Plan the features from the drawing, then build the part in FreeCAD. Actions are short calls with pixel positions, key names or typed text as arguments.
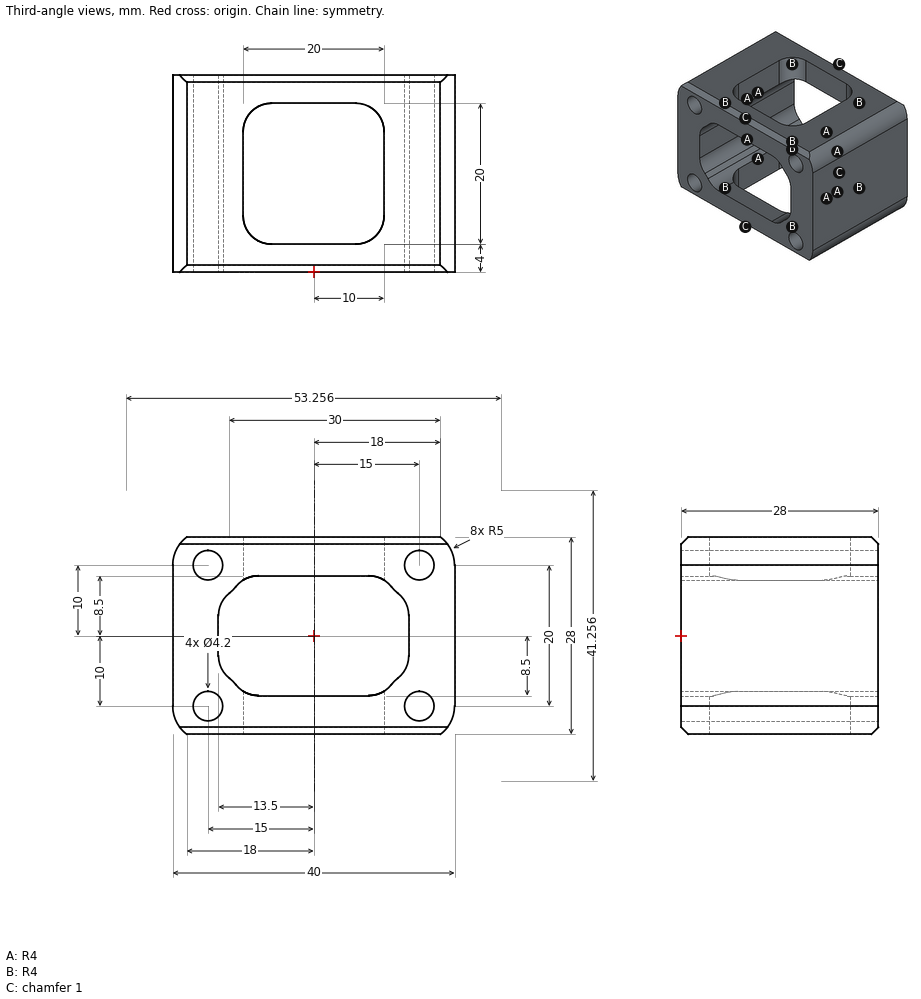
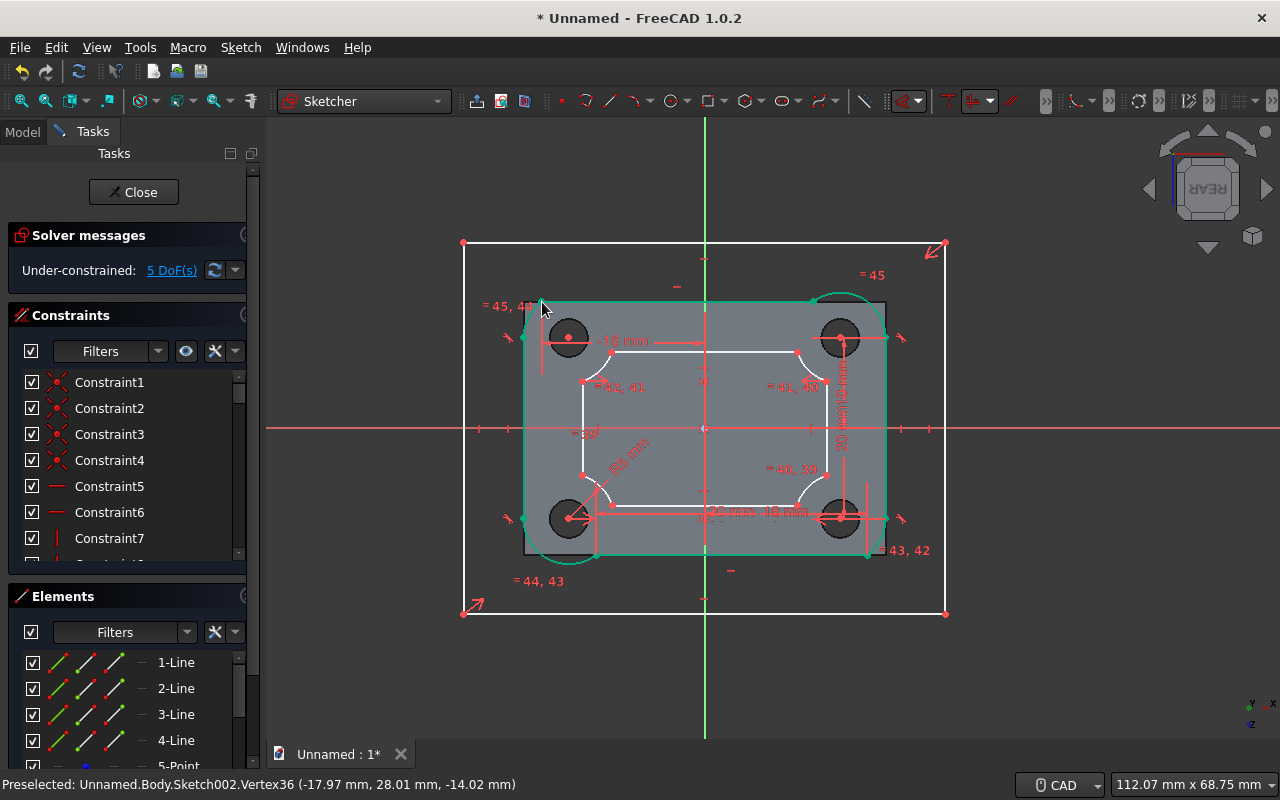
click(612, 506)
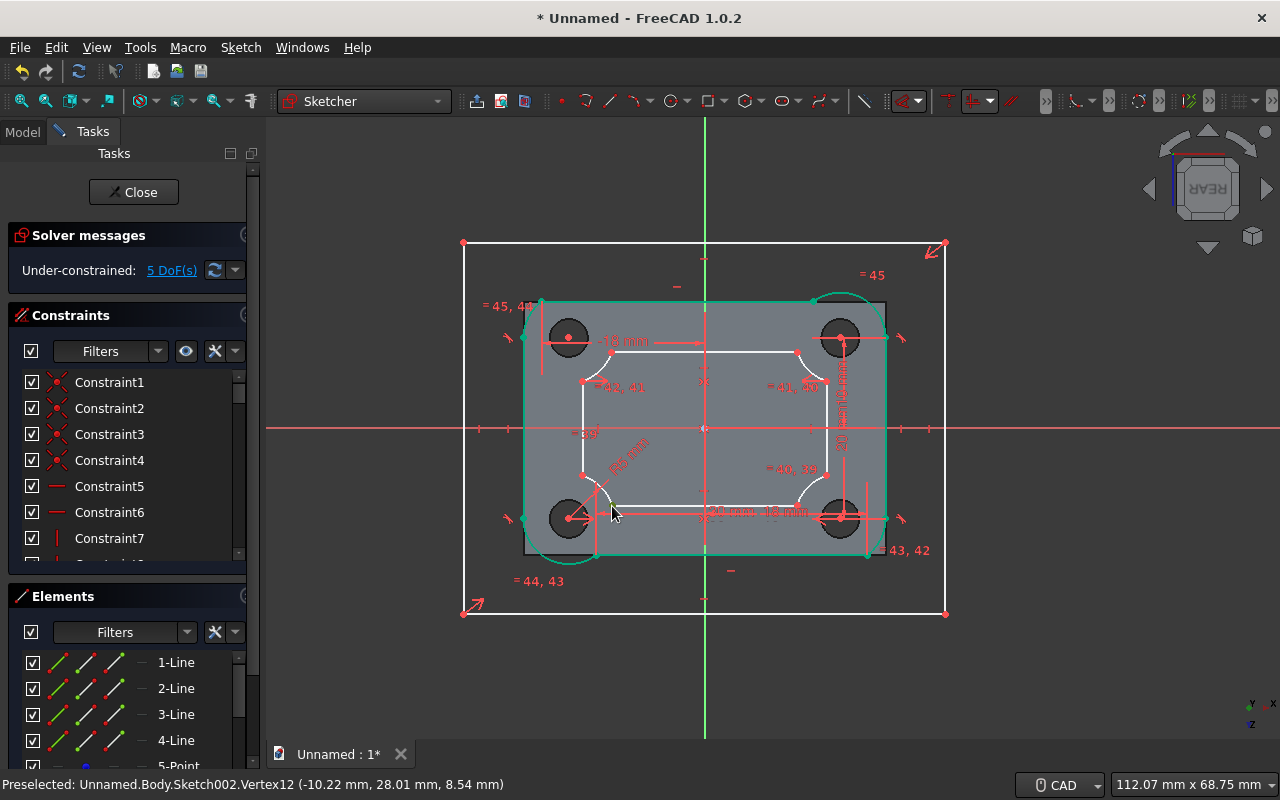
click(920, 102)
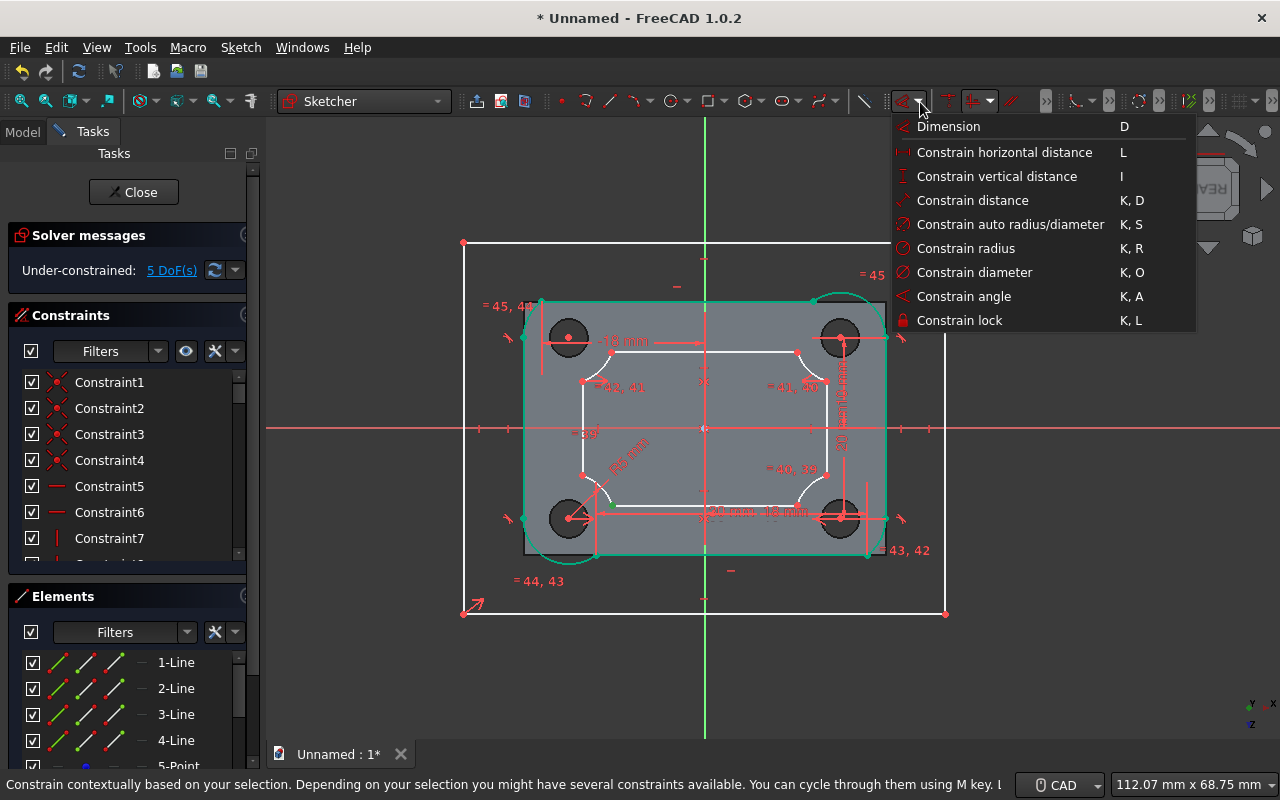
click(1044, 176)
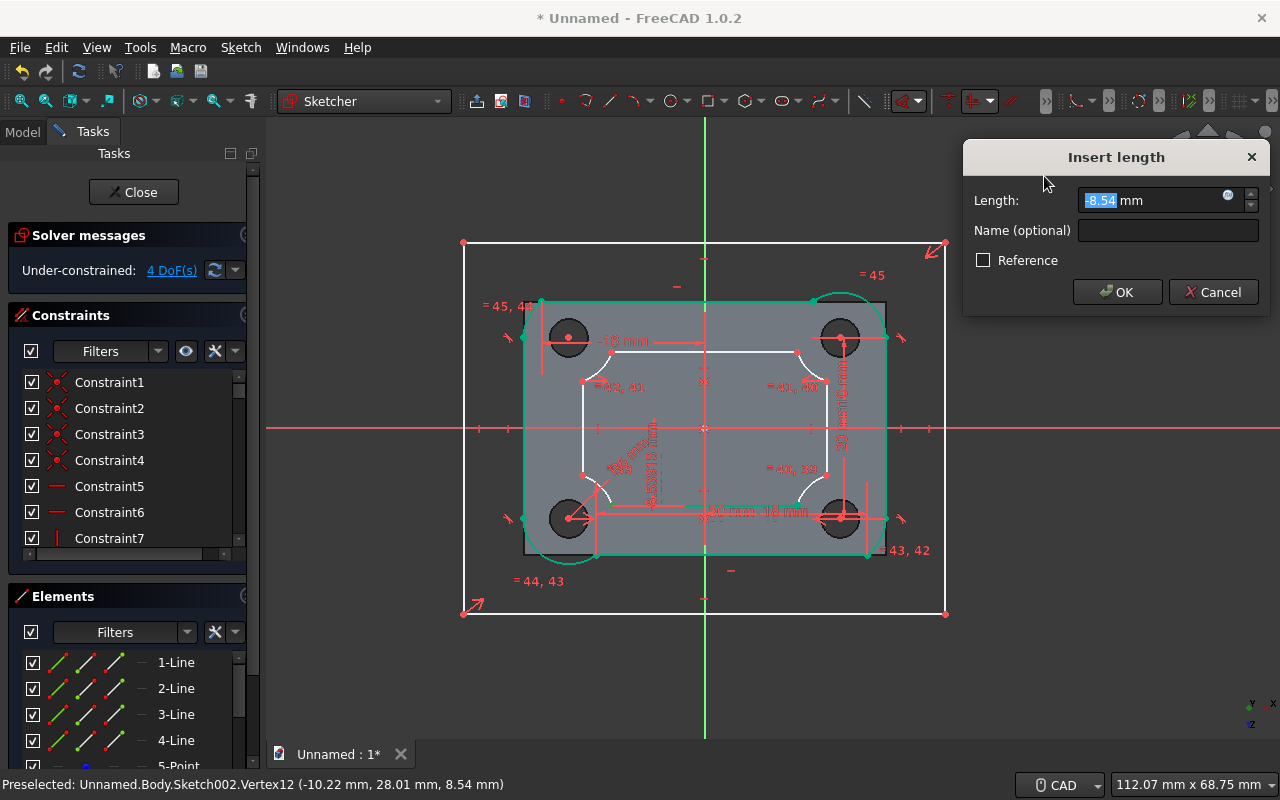
text(-8.5)
key(Return)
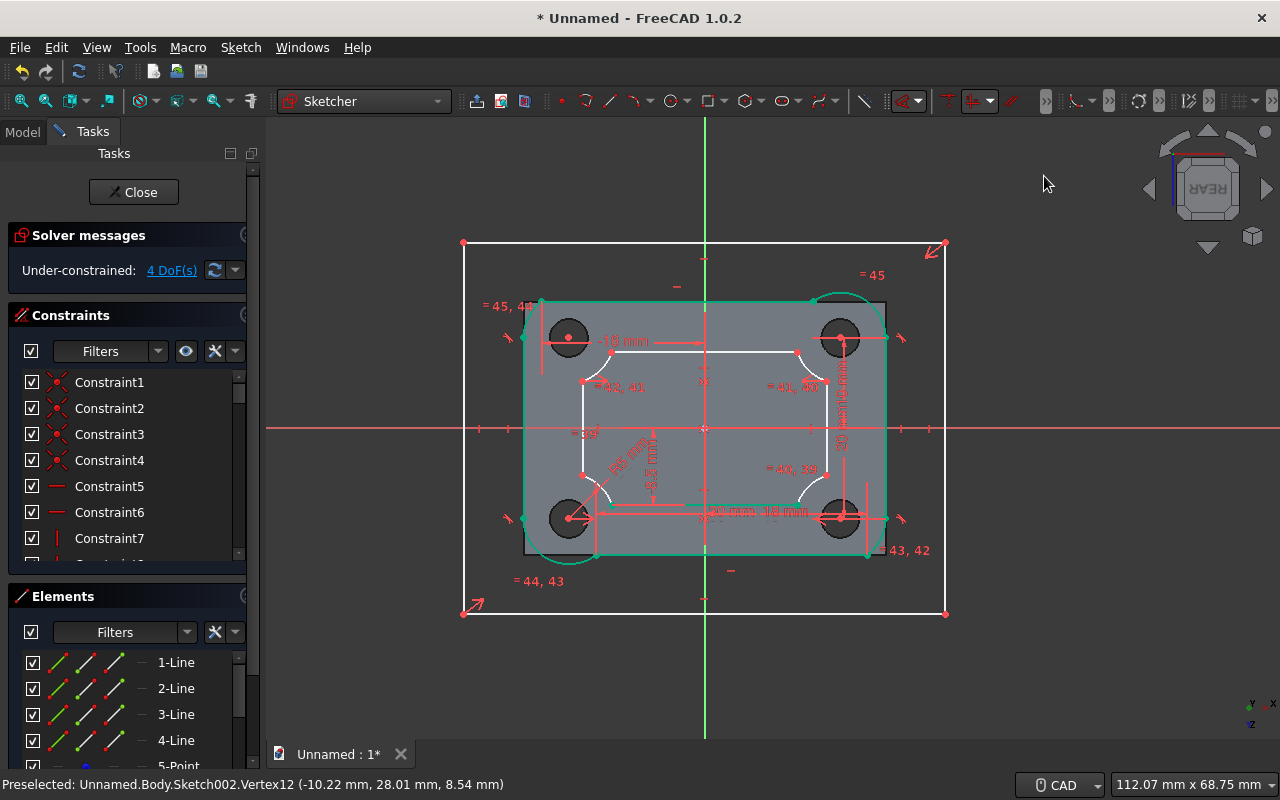
click(797, 352)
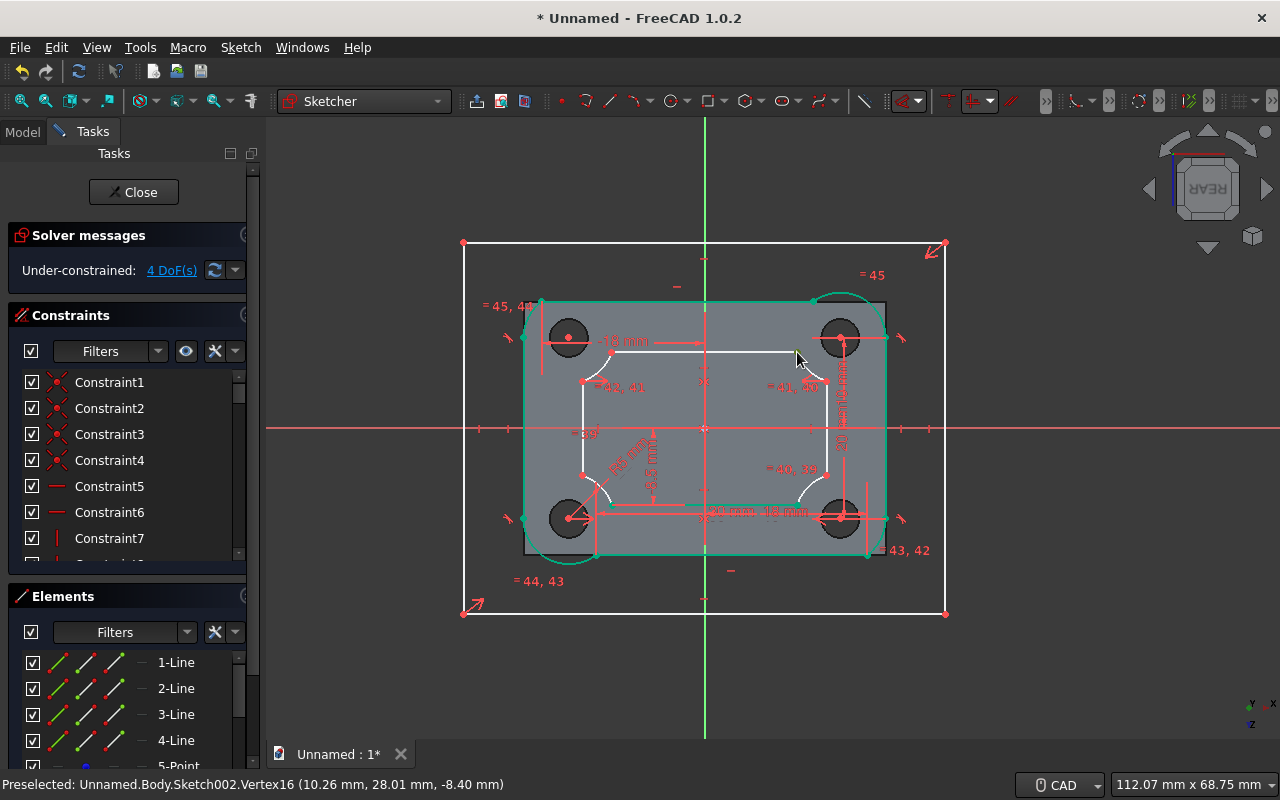
key(i)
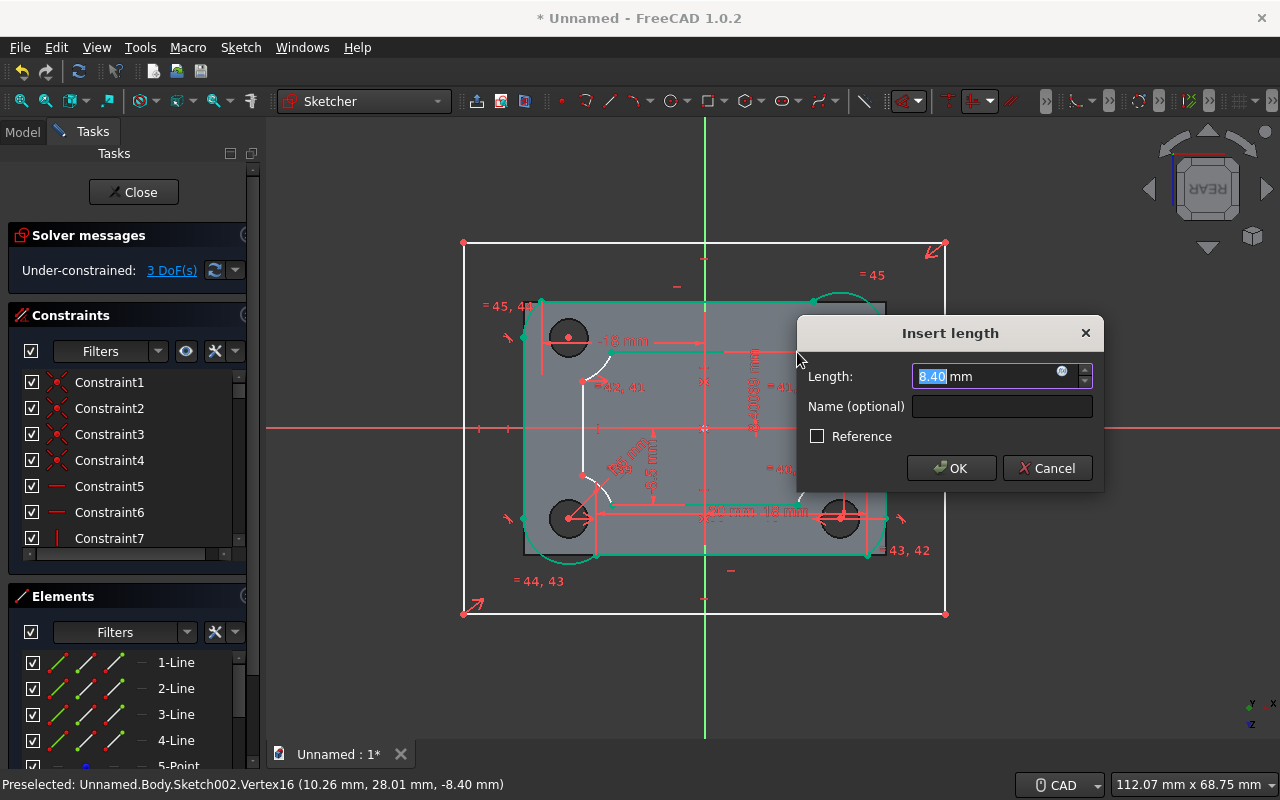
text(8.5)
key(Return)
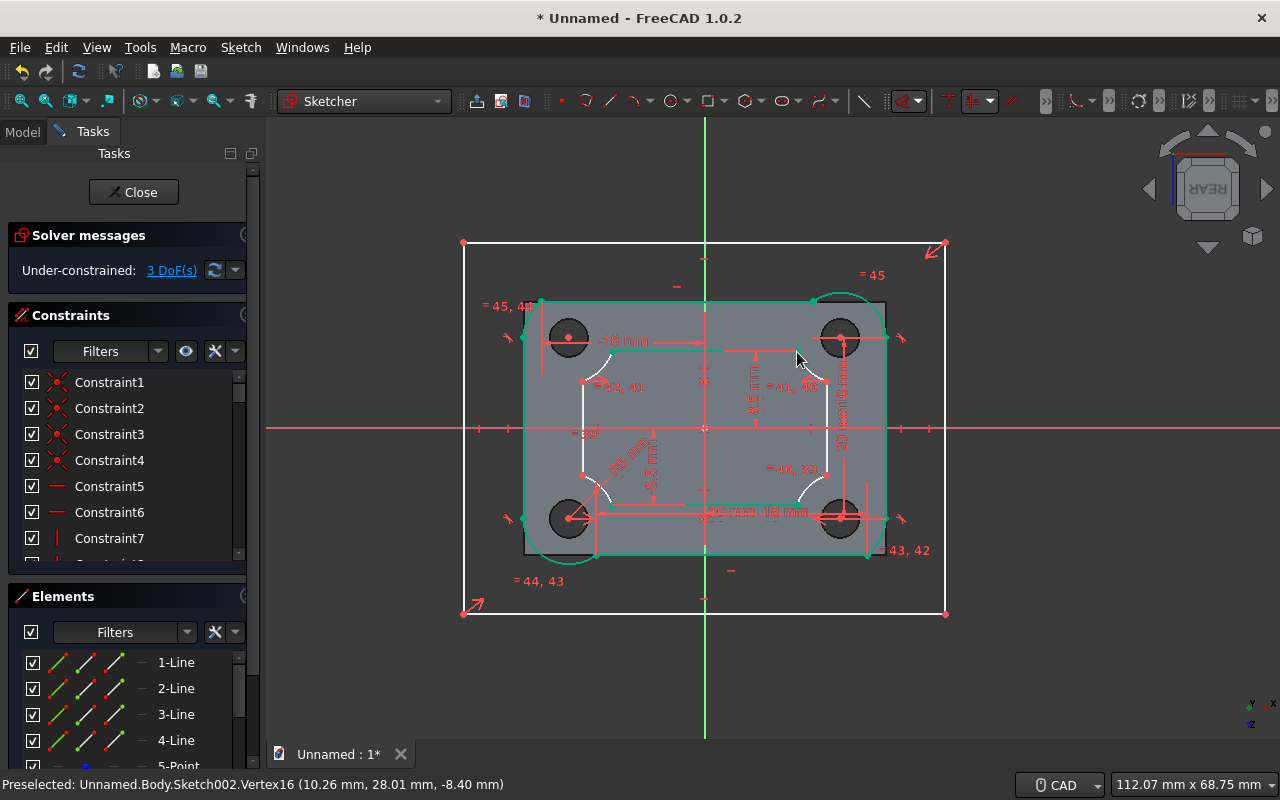
click(583, 381)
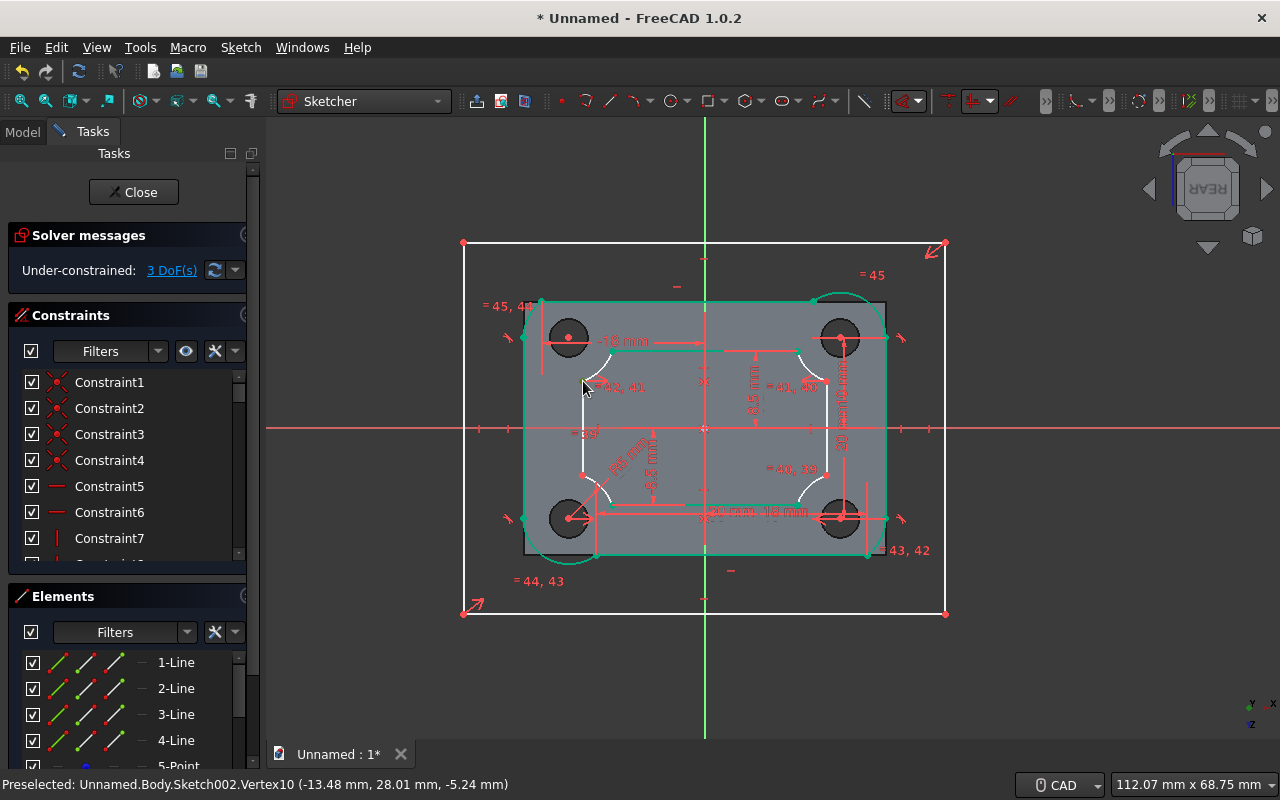
key(l)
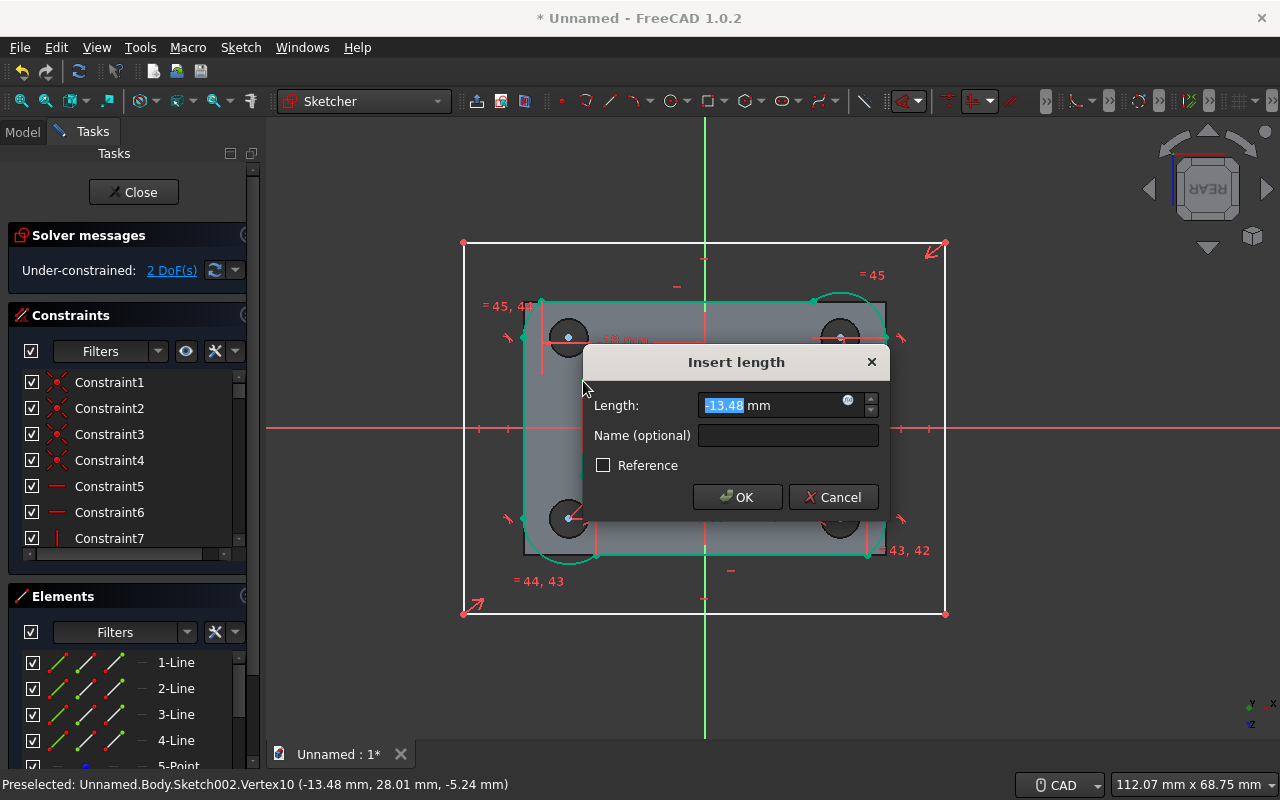
text(-13.5)
key(Return)